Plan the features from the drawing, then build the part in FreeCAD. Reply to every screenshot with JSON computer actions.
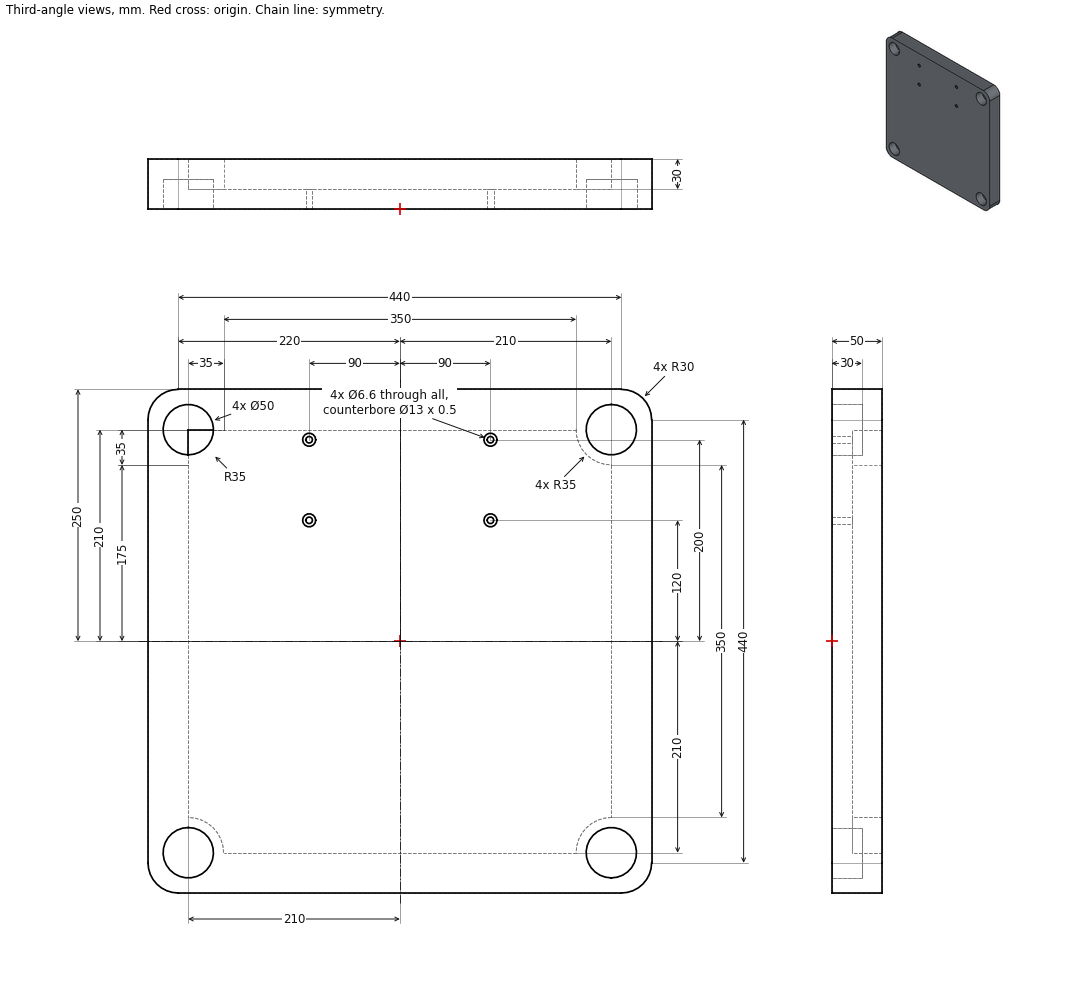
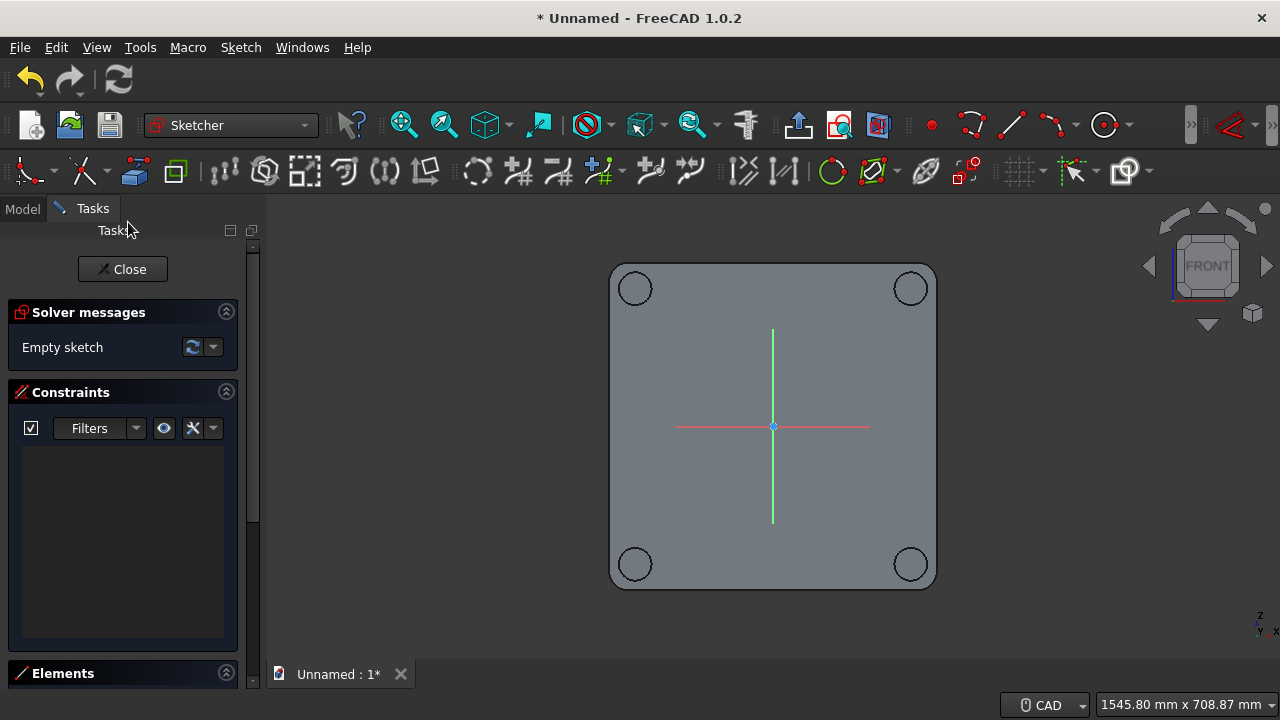
{"action": "scroll", "coordinate": [829, 305], "scroll_direction": "up", "scroll_amount": 4}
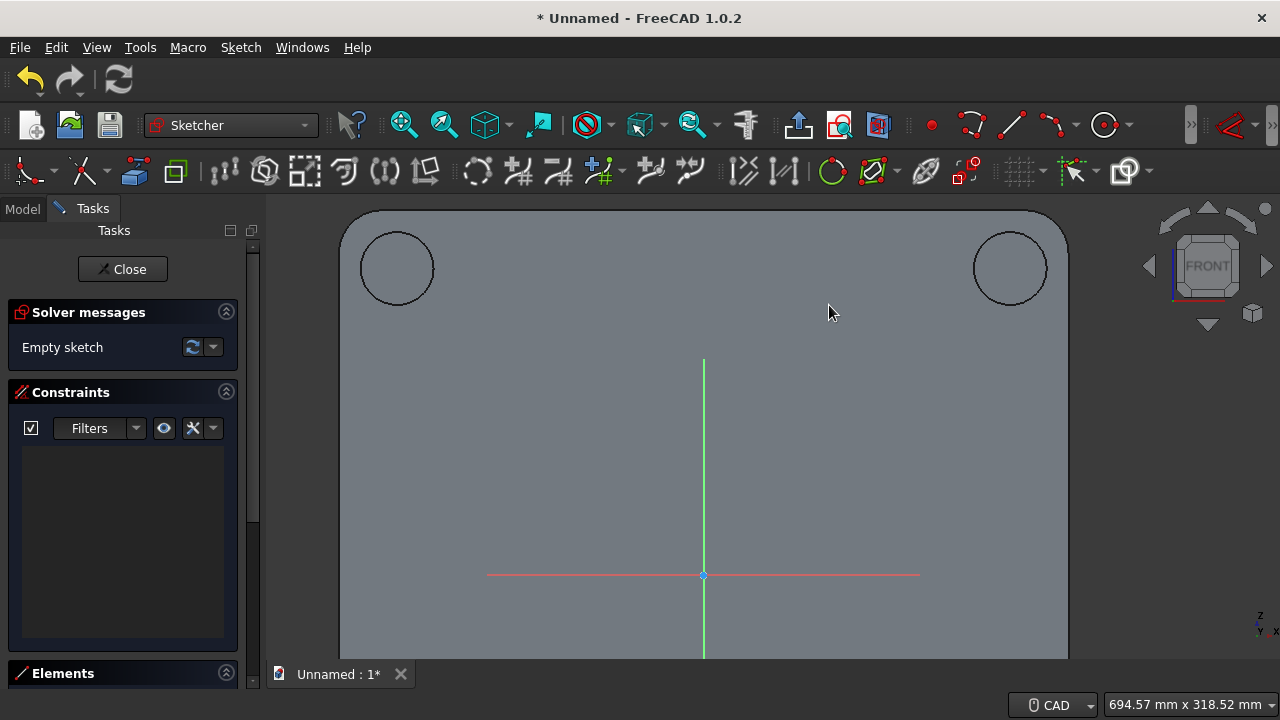
{"action": "key", "text": "g c"}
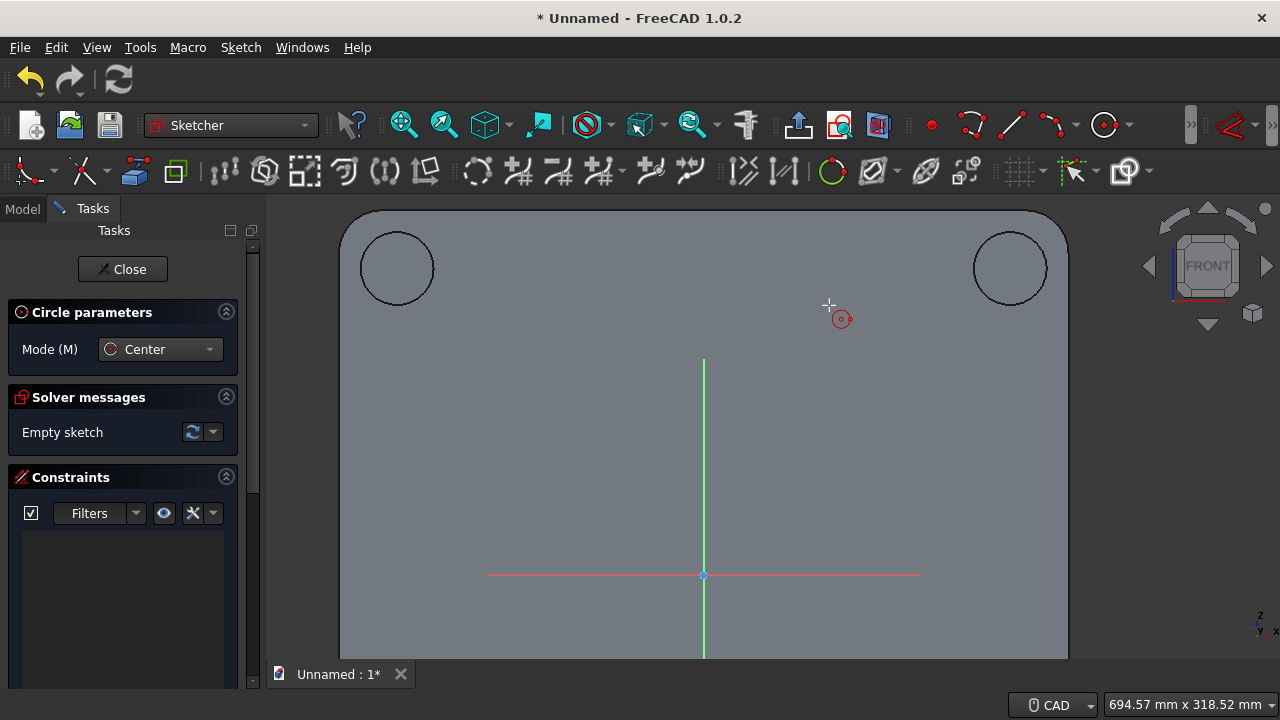
{"action": "scroll", "coordinate": [835, 283], "scroll_direction": "up", "scroll_amount": 8}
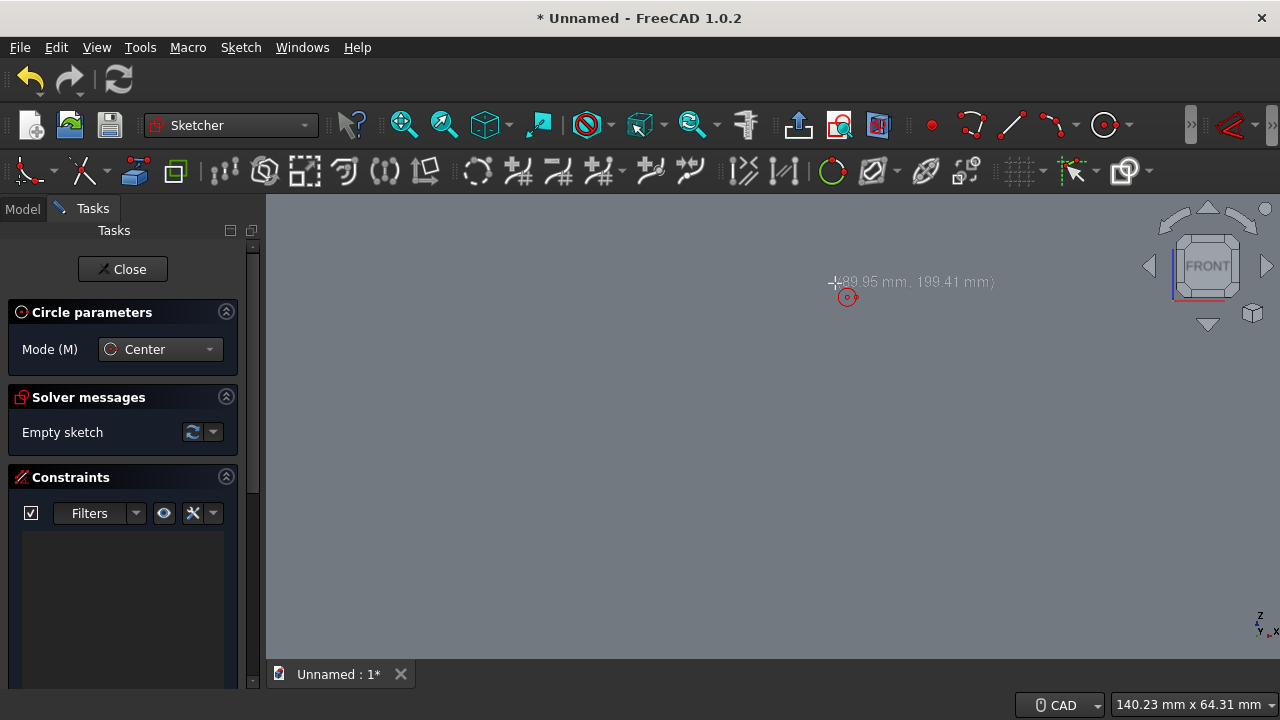
{"action": "scroll", "coordinate": [837, 283], "scroll_direction": "down", "scroll_amount": 8}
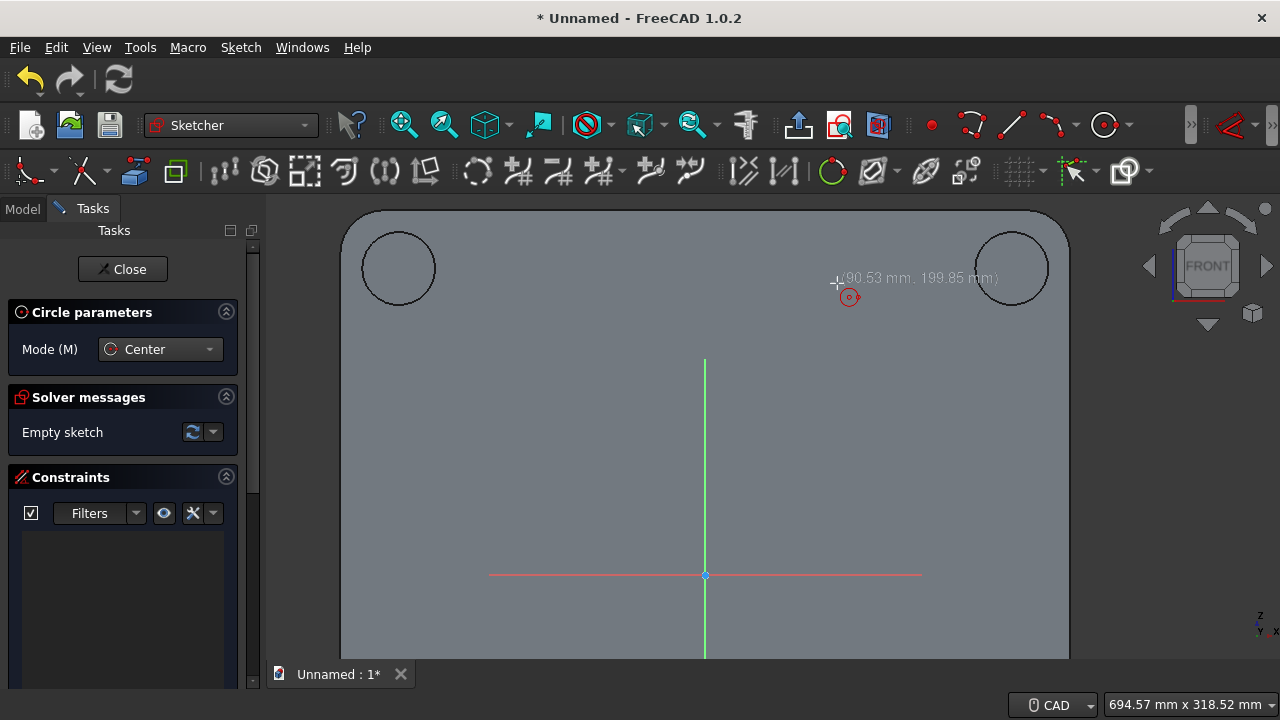
{"action": "left_click", "coordinate": [837, 283]}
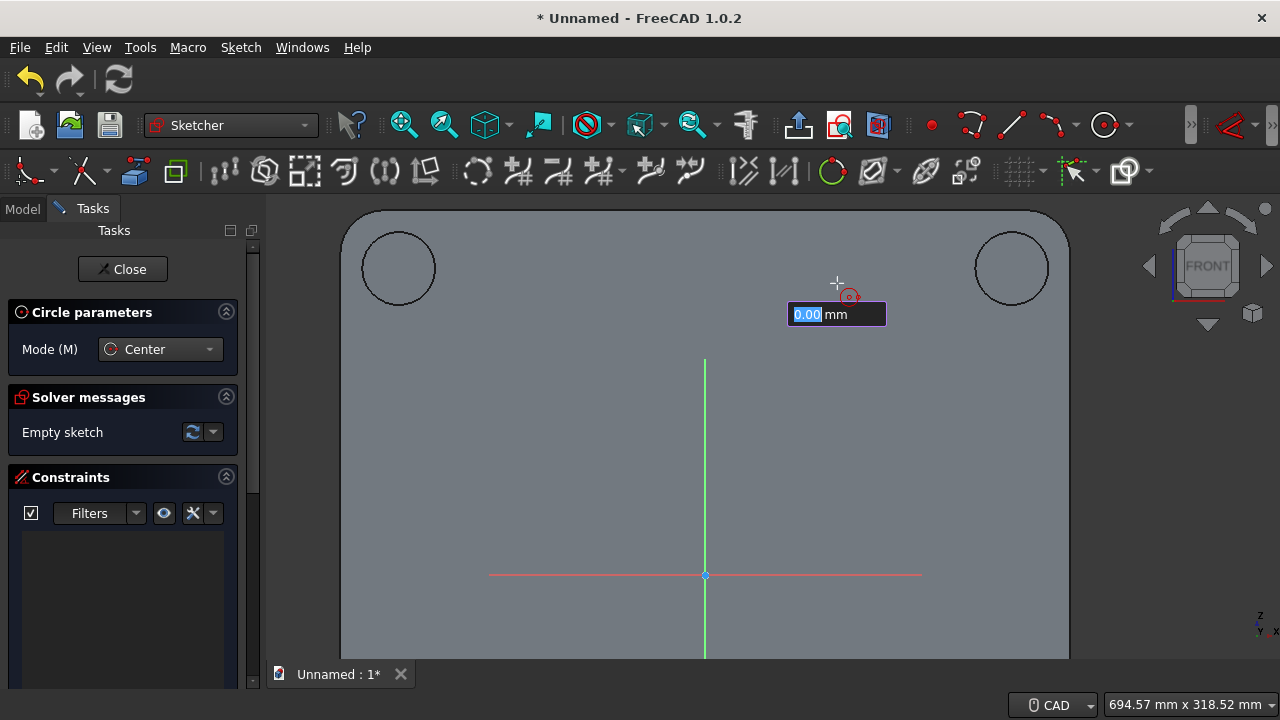
{"action": "scroll", "coordinate": [840, 280], "scroll_direction": "up", "scroll_amount": 6}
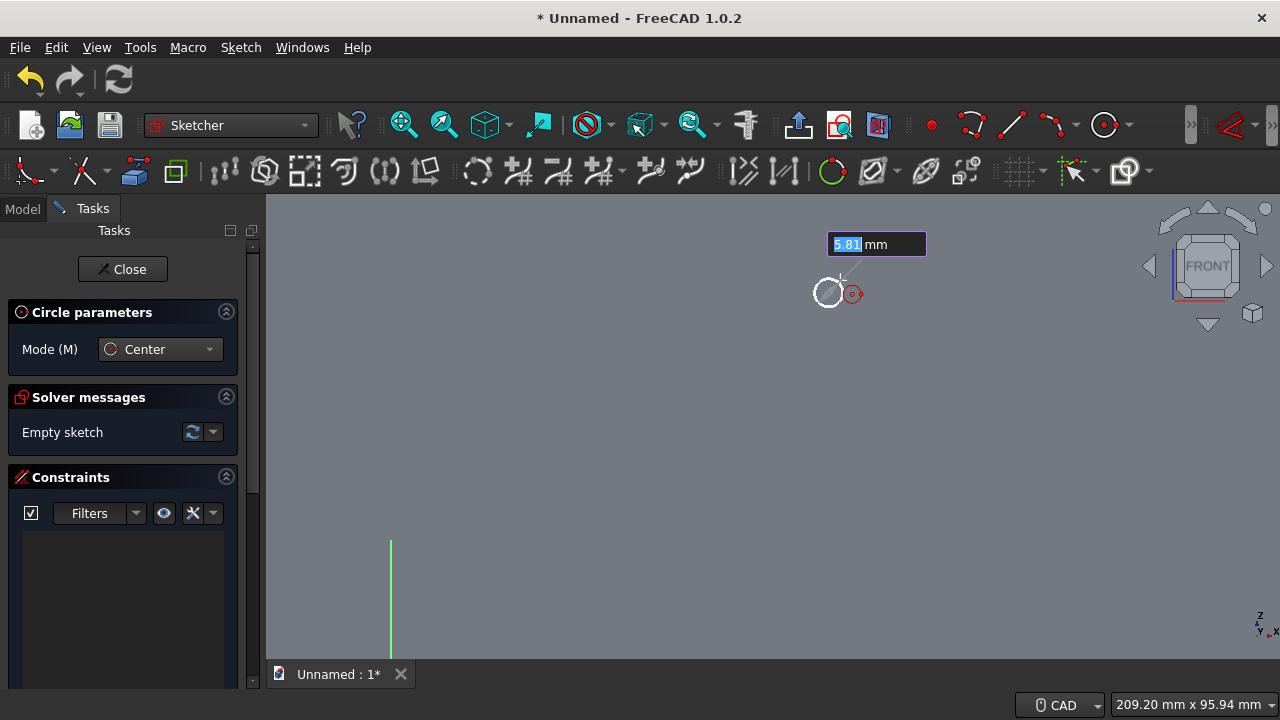
{"action": "left_click", "coordinate": [839, 279]}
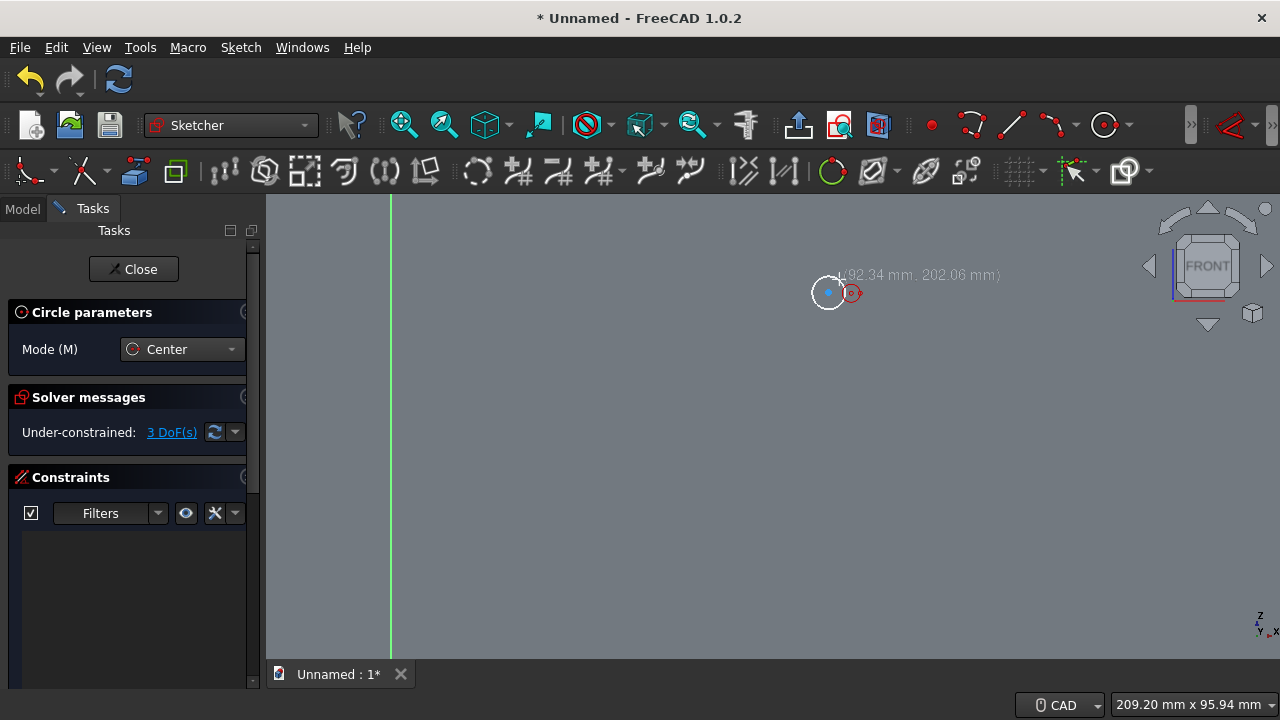
{"action": "scroll", "coordinate": [839, 280], "scroll_direction": "down", "scroll_amount": 6}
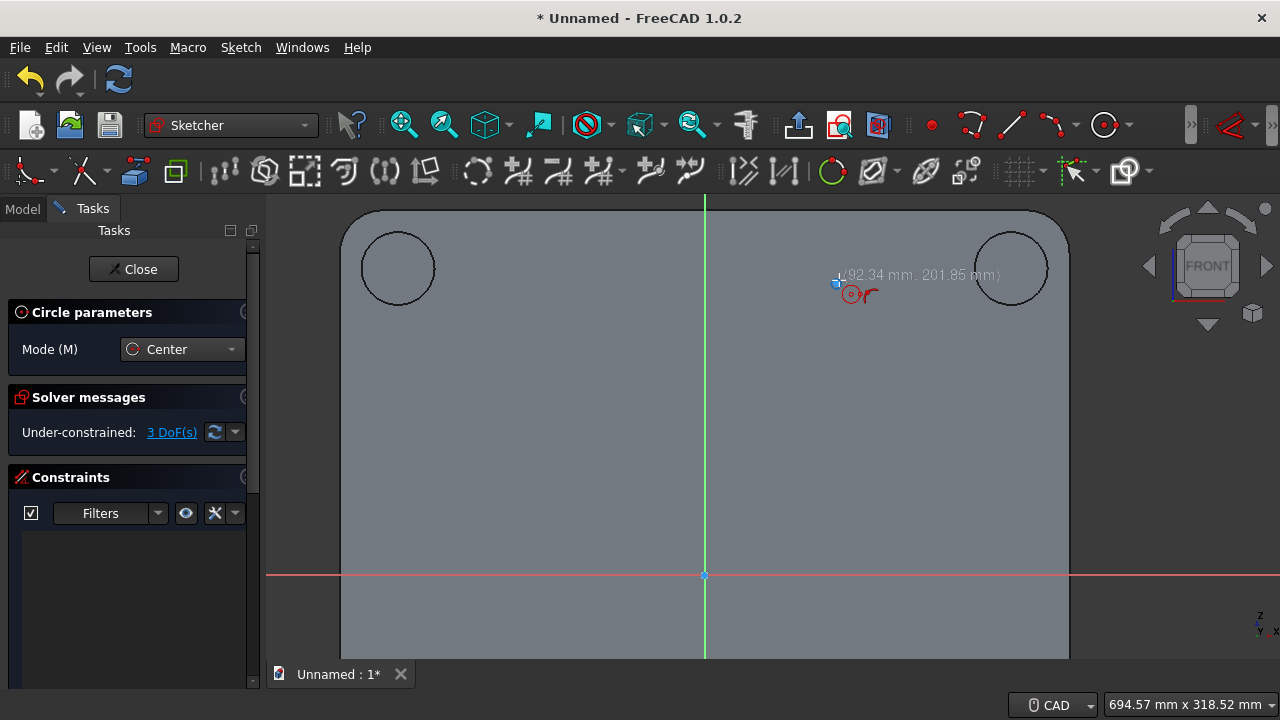
{"action": "scroll", "coordinate": [573, 283], "scroll_direction": "up", "scroll_amount": 8}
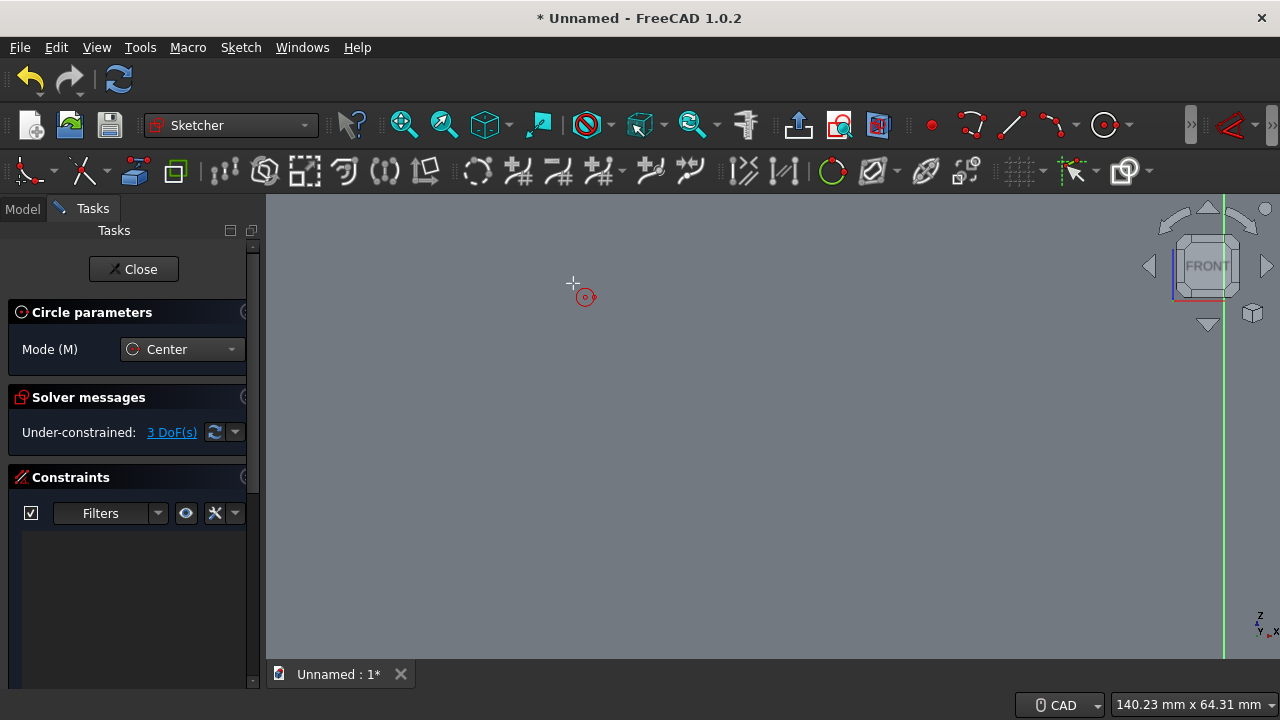
{"action": "scroll", "coordinate": [573, 283], "scroll_direction": "down", "scroll_amount": 8}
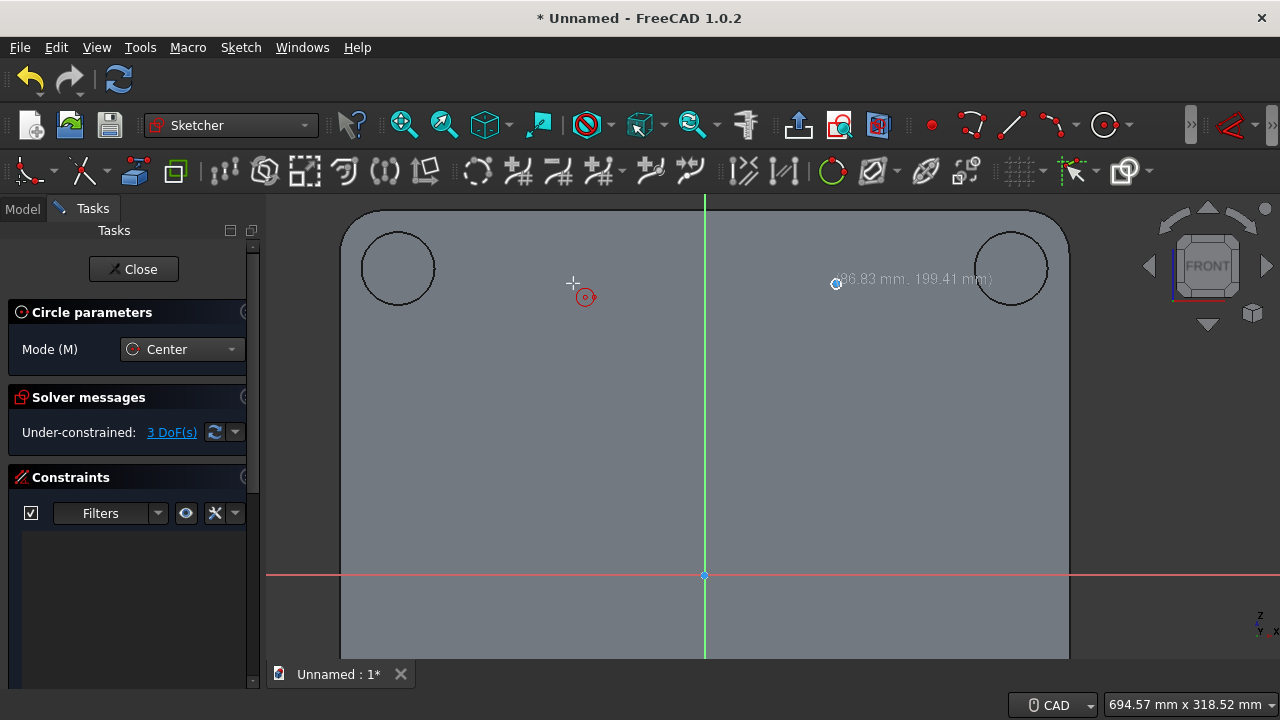
{"action": "left_click", "coordinate": [573, 283]}